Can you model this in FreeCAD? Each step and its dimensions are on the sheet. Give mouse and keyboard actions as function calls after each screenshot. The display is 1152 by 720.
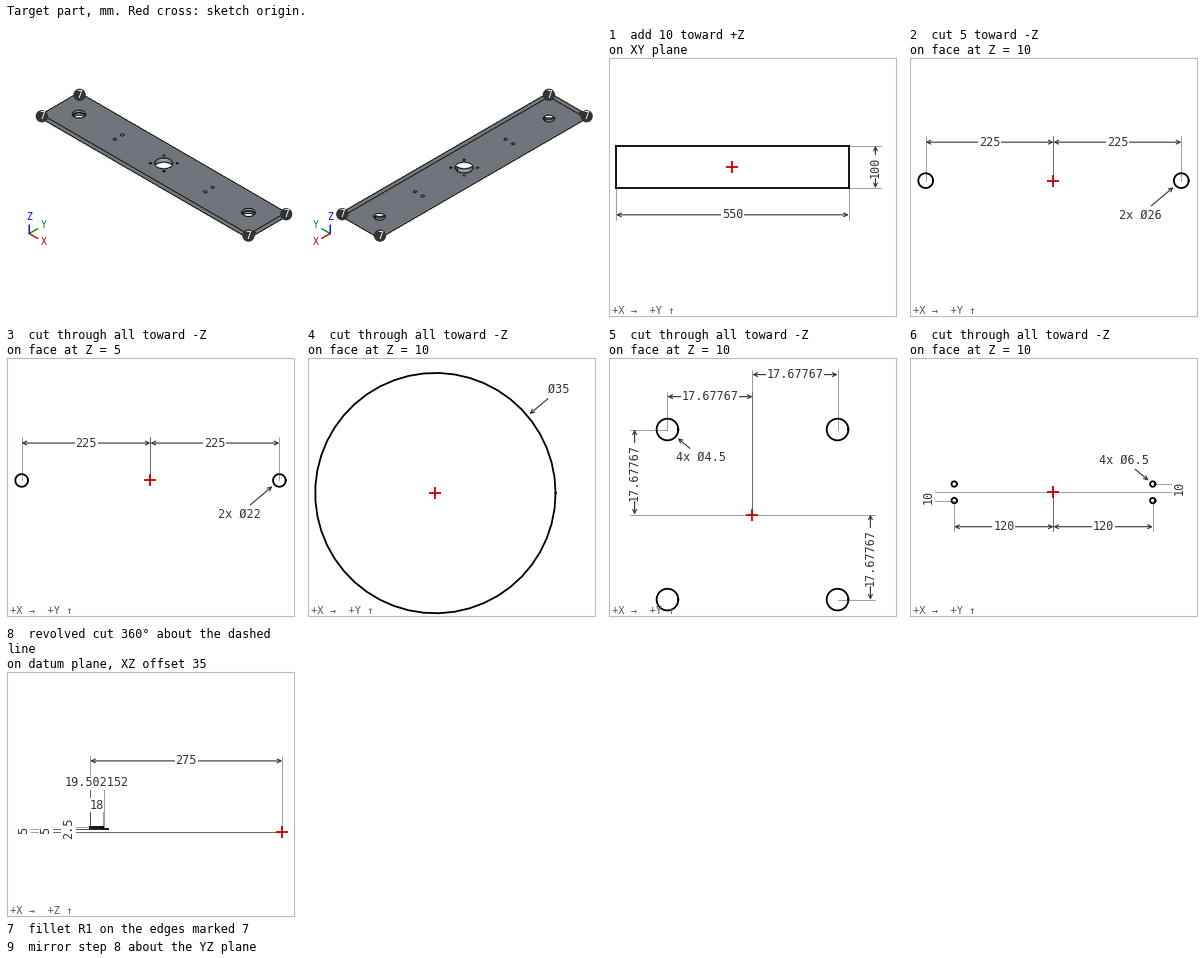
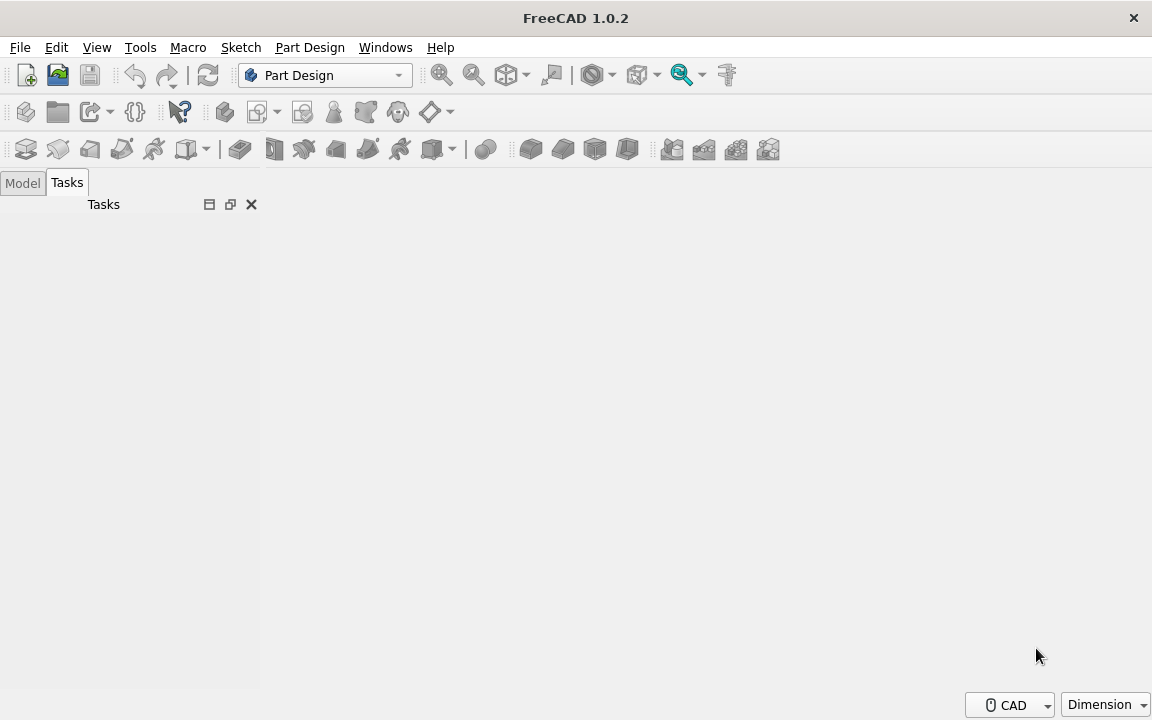
click(532, 76)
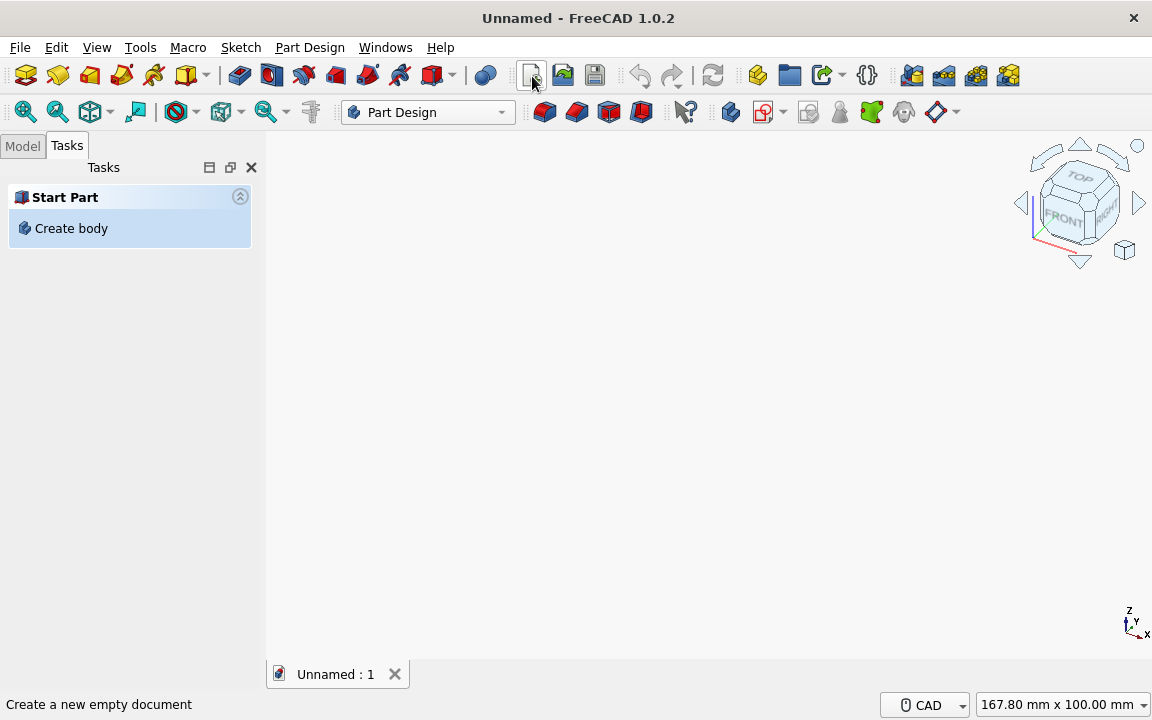
click(764, 112)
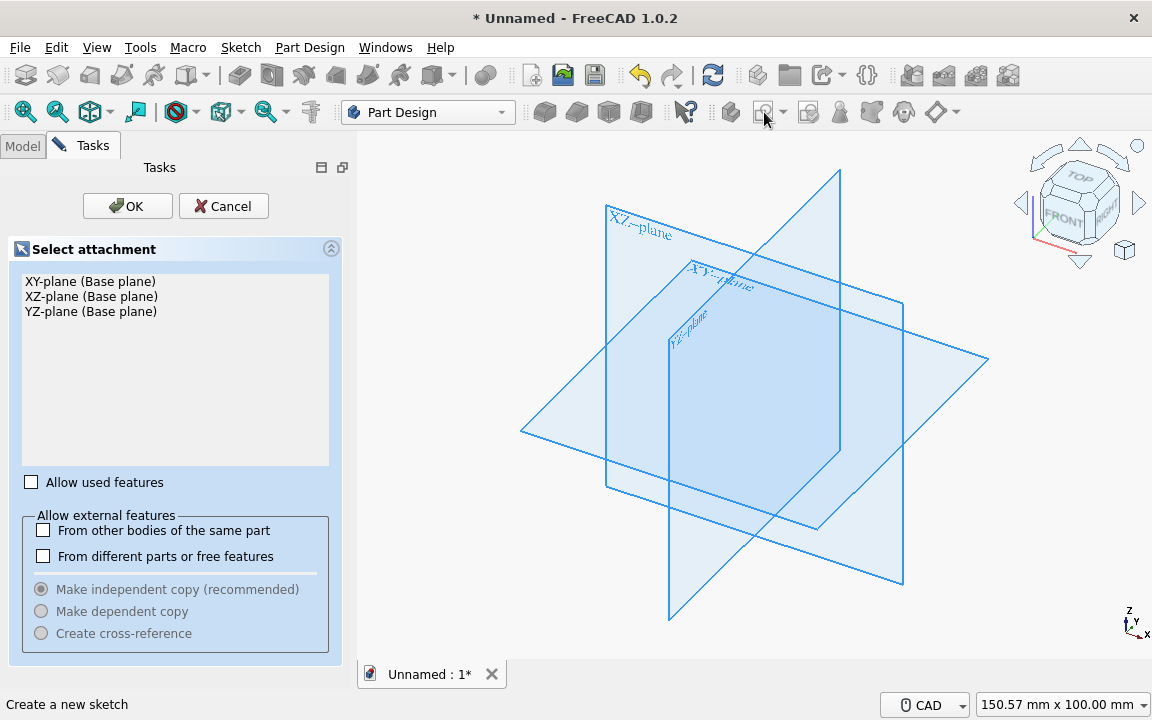
click(82, 282)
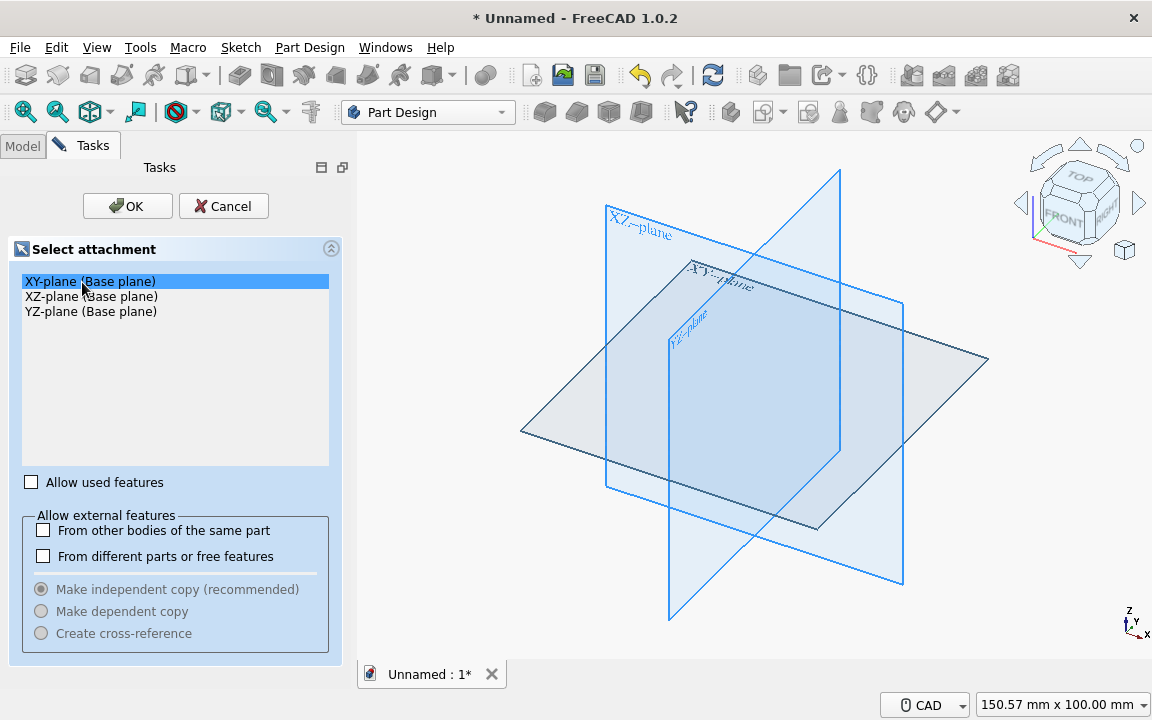
click(128, 206)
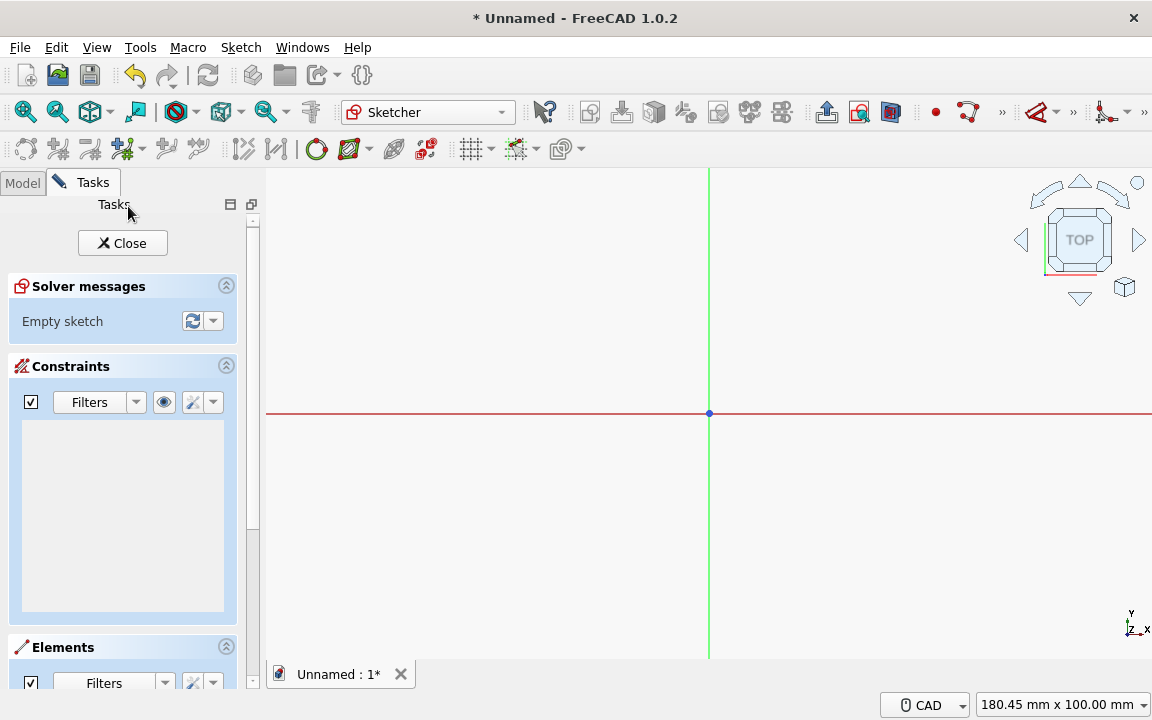
scroll(627, 414, down, 9)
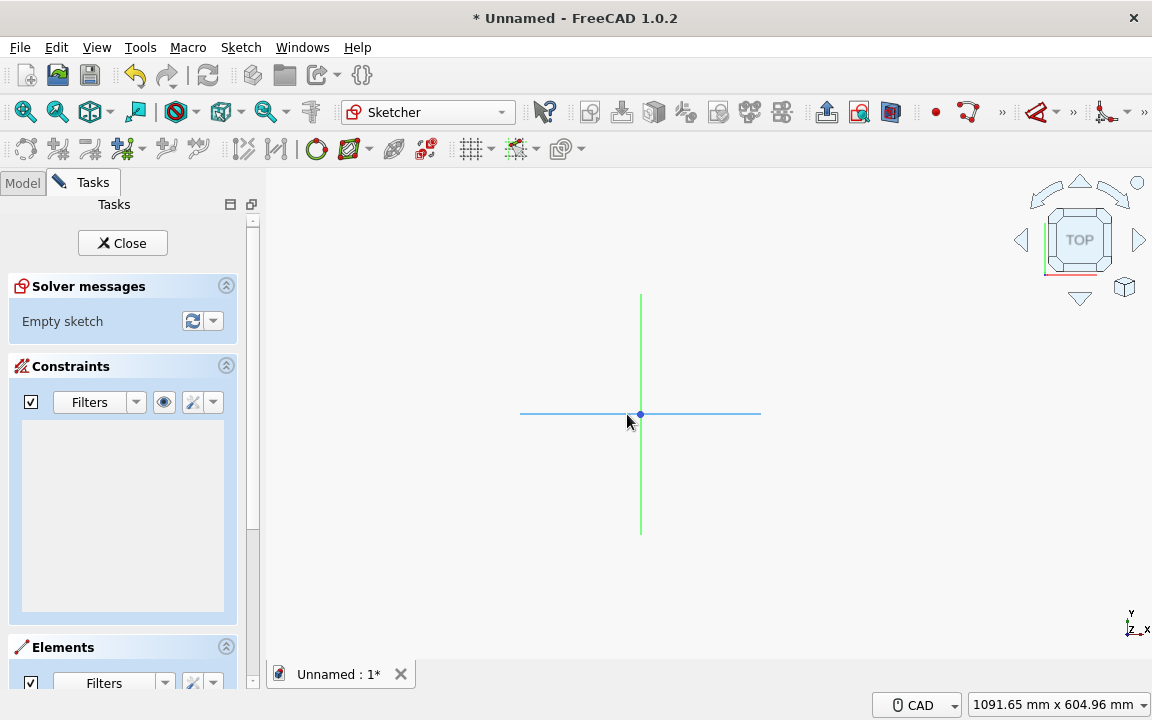
key(g)
key(v)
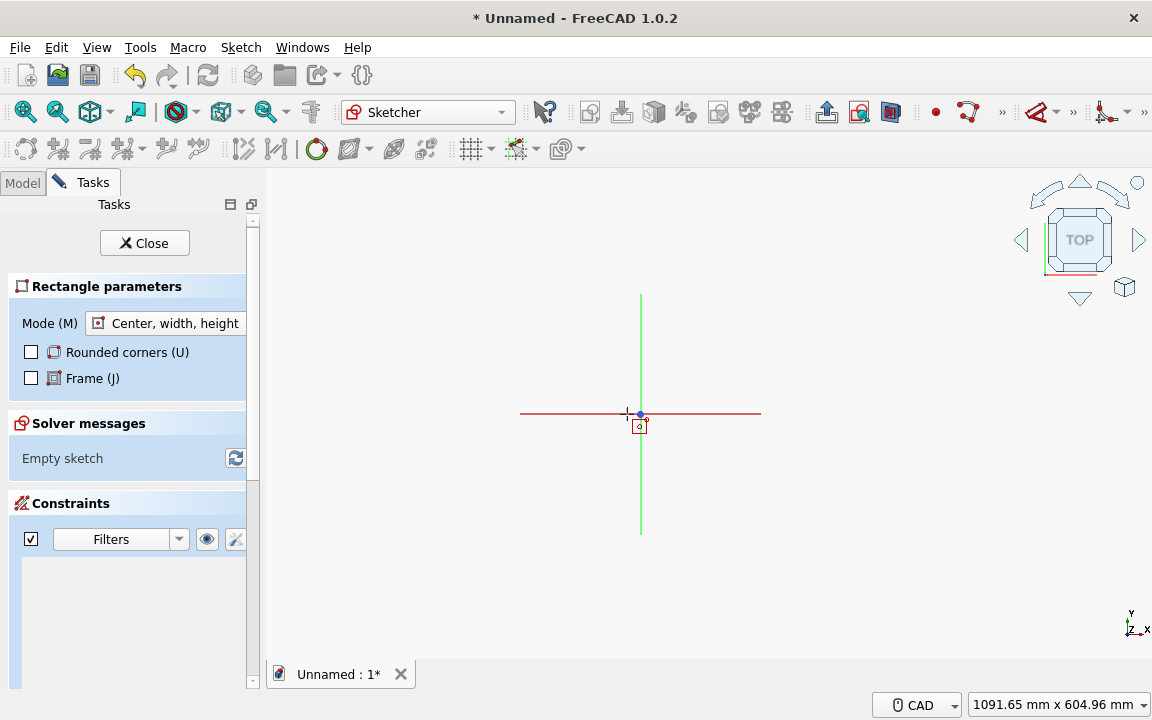
click(641, 414)
move(864, 374)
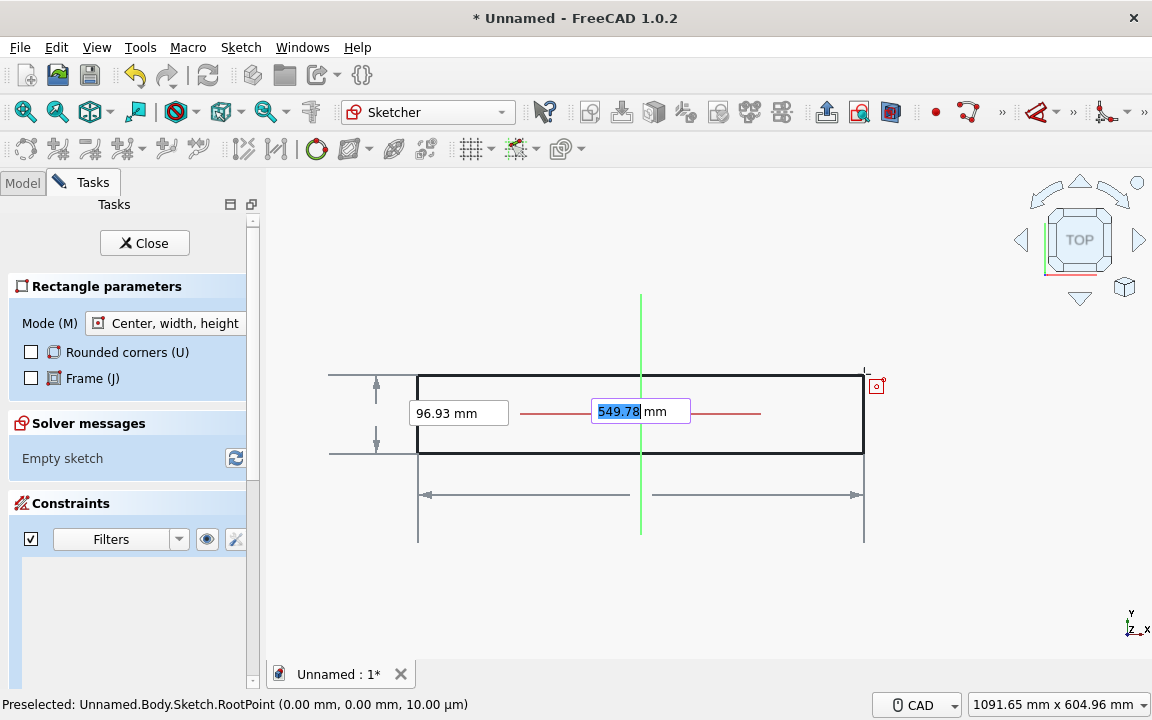
text(550)
key(Tab)
text(100)
key(Return)
key(Escape)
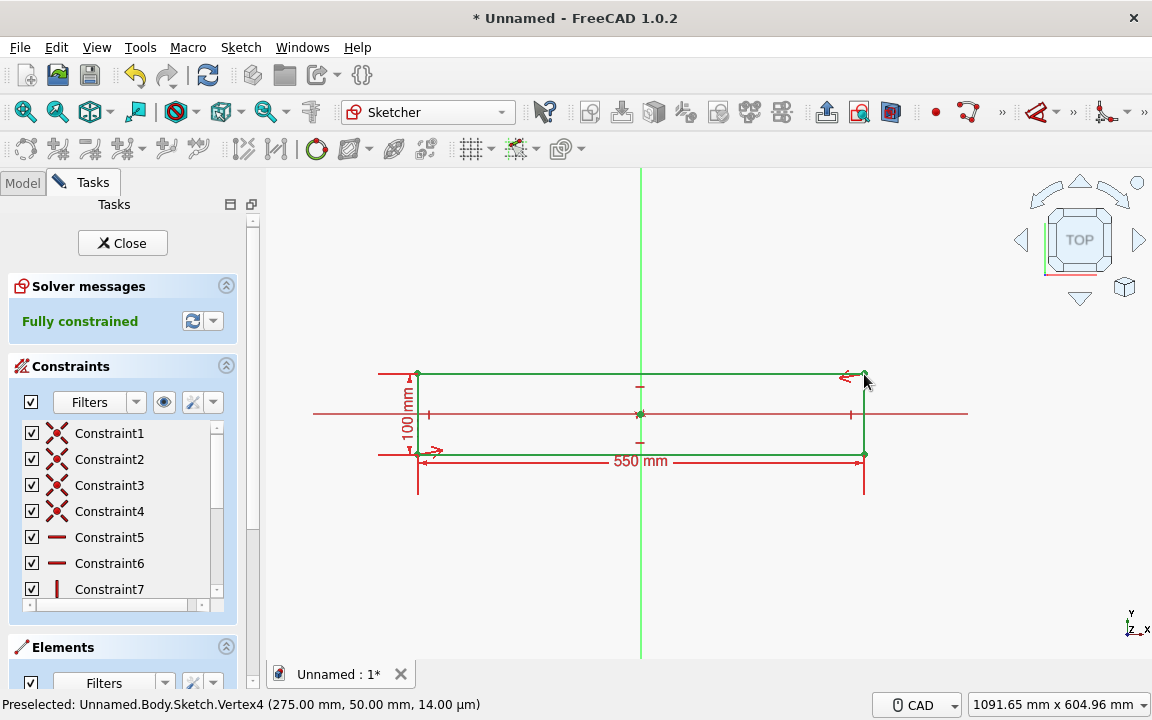
click(123, 243)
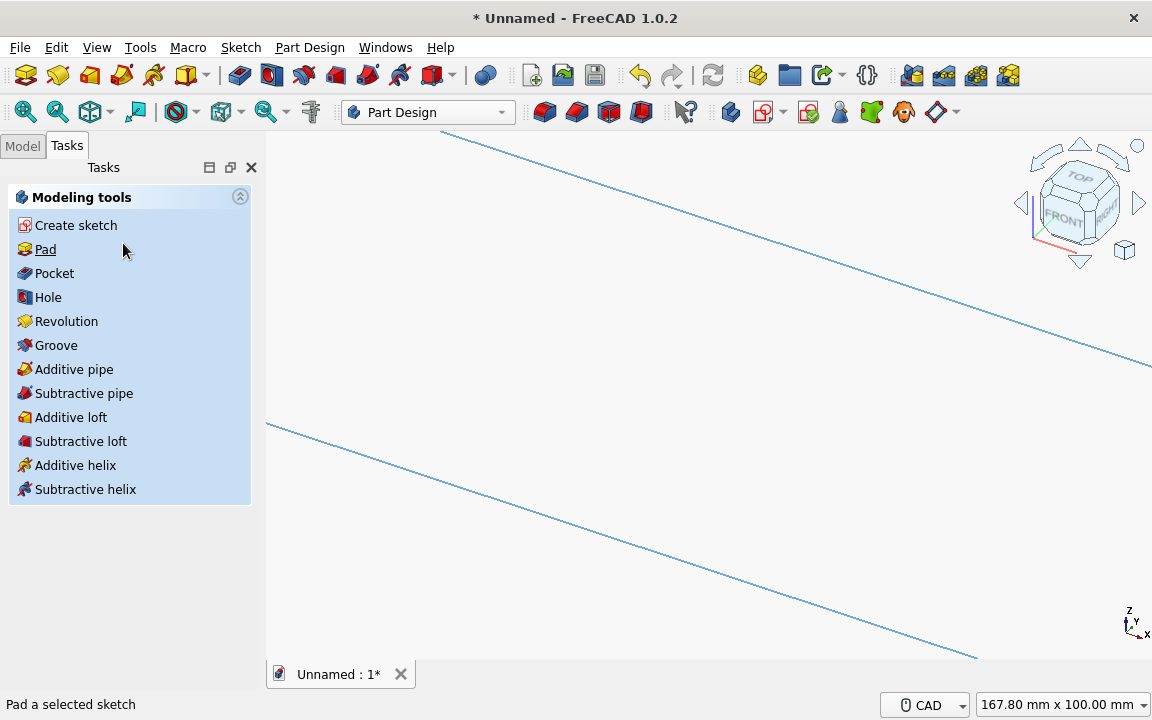
click(26, 76)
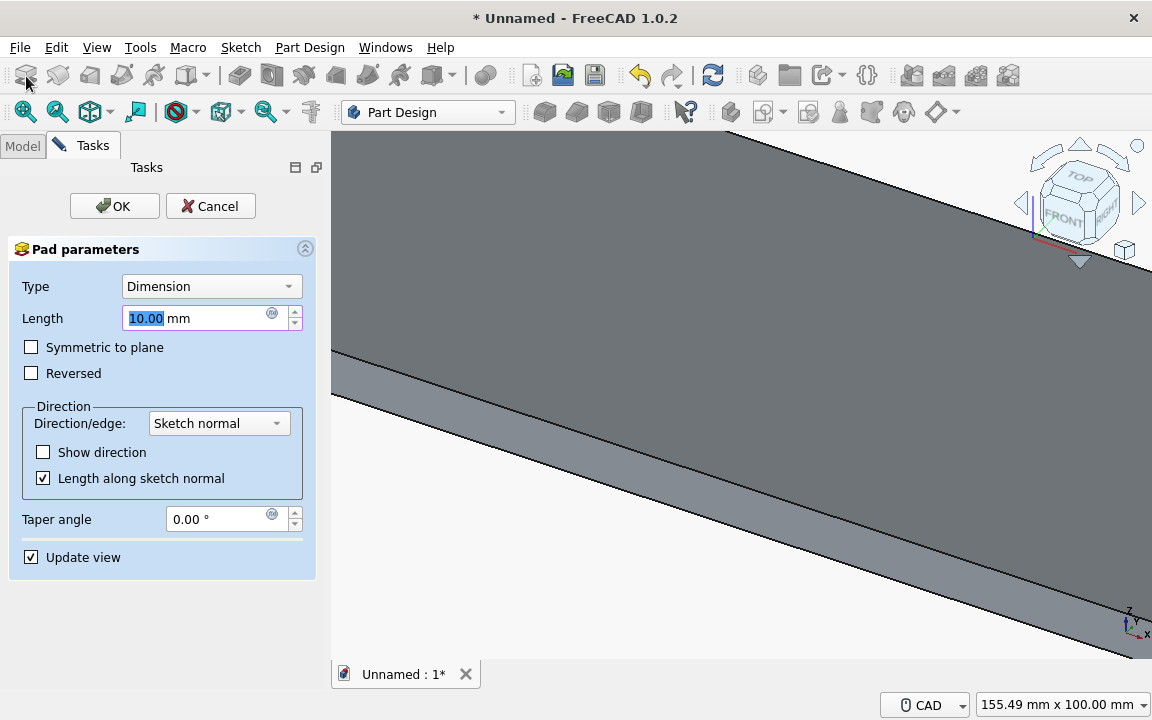
text(10)
key(Tab)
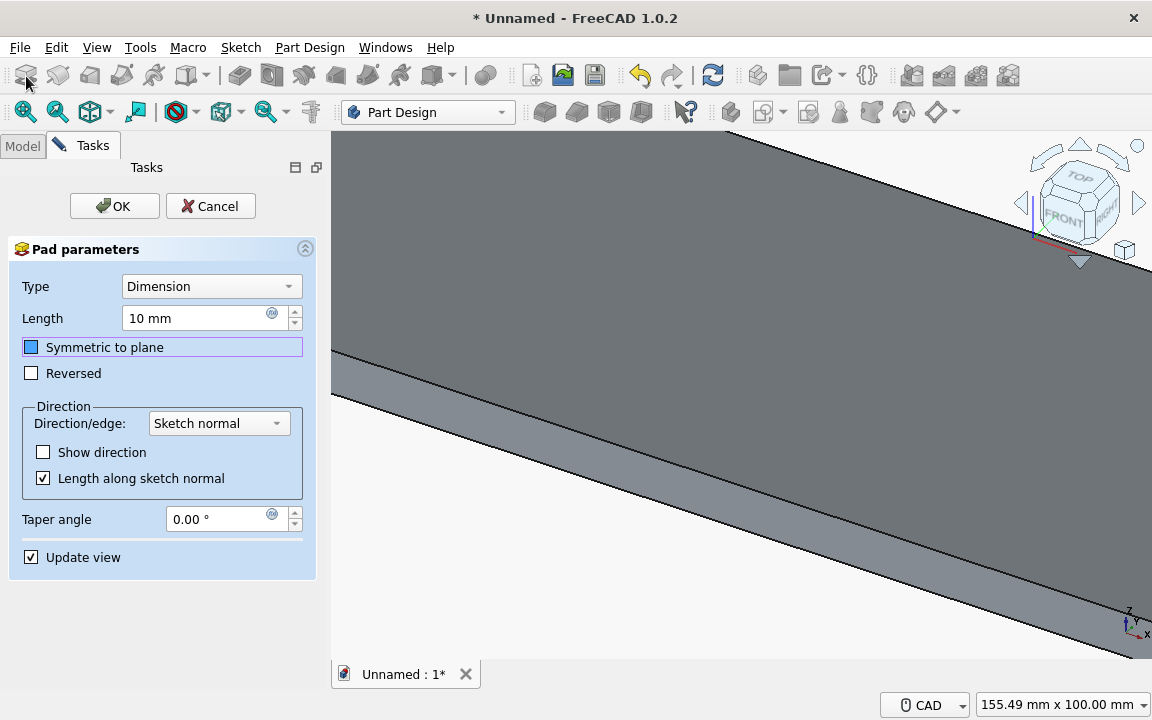
click(115, 206)